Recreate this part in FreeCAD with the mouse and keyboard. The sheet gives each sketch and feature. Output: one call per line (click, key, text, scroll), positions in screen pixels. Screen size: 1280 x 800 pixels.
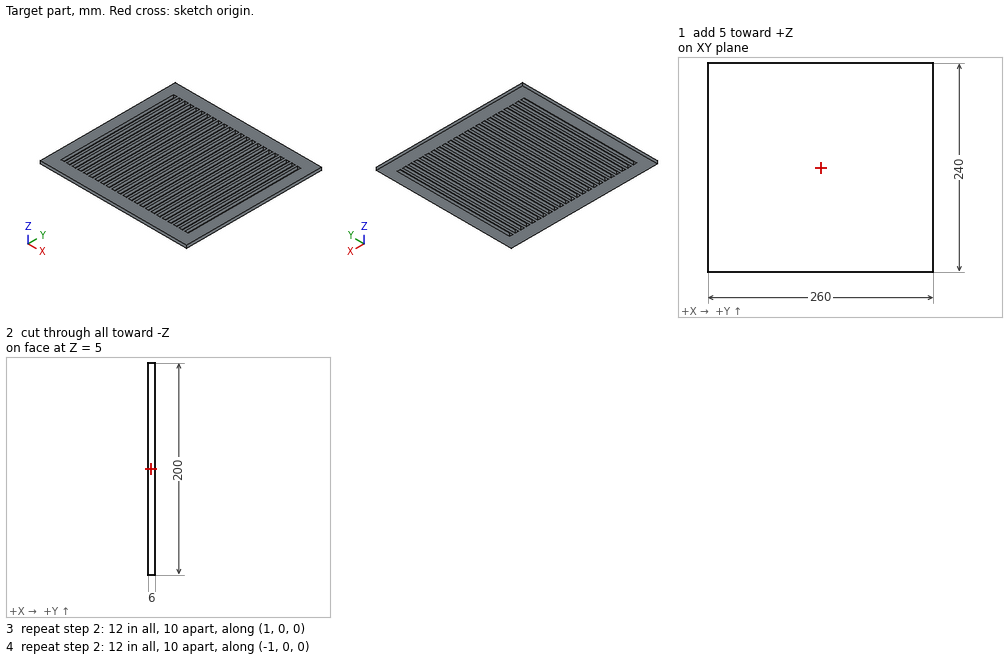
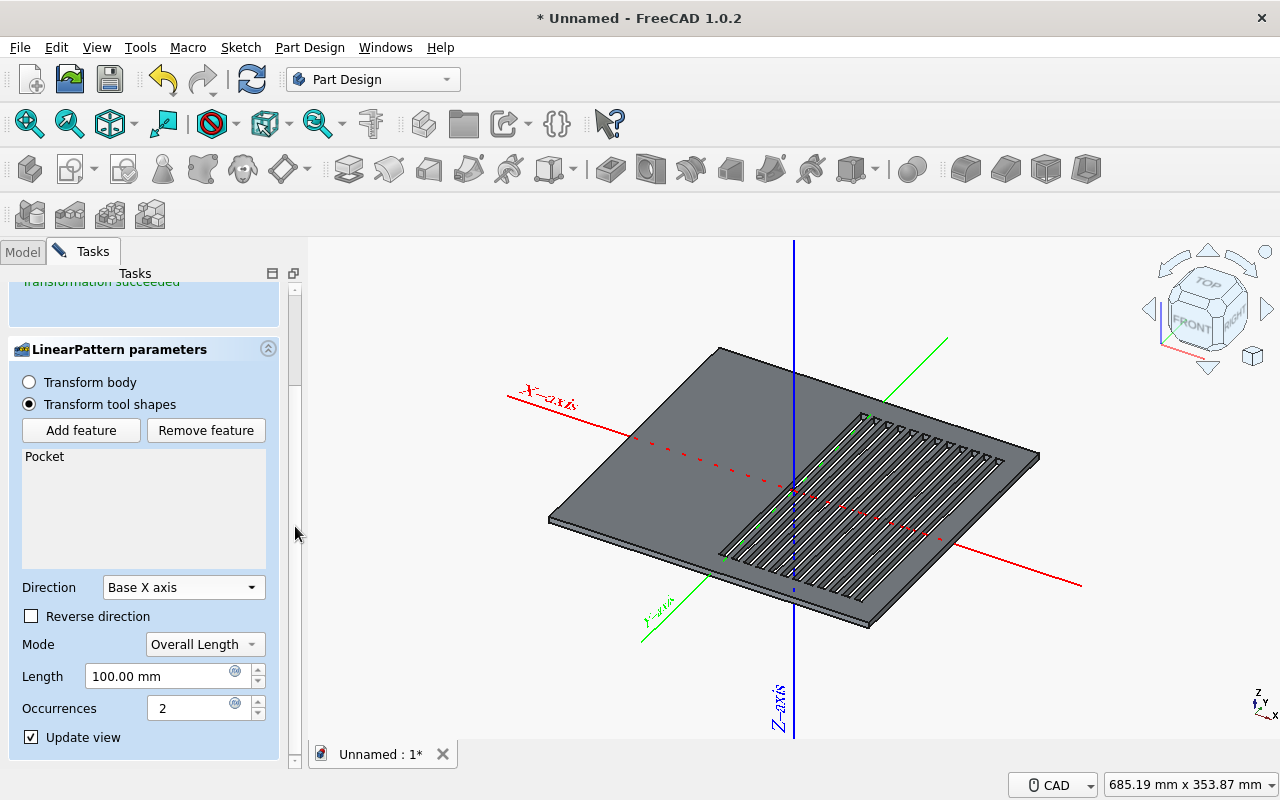
click(206, 644)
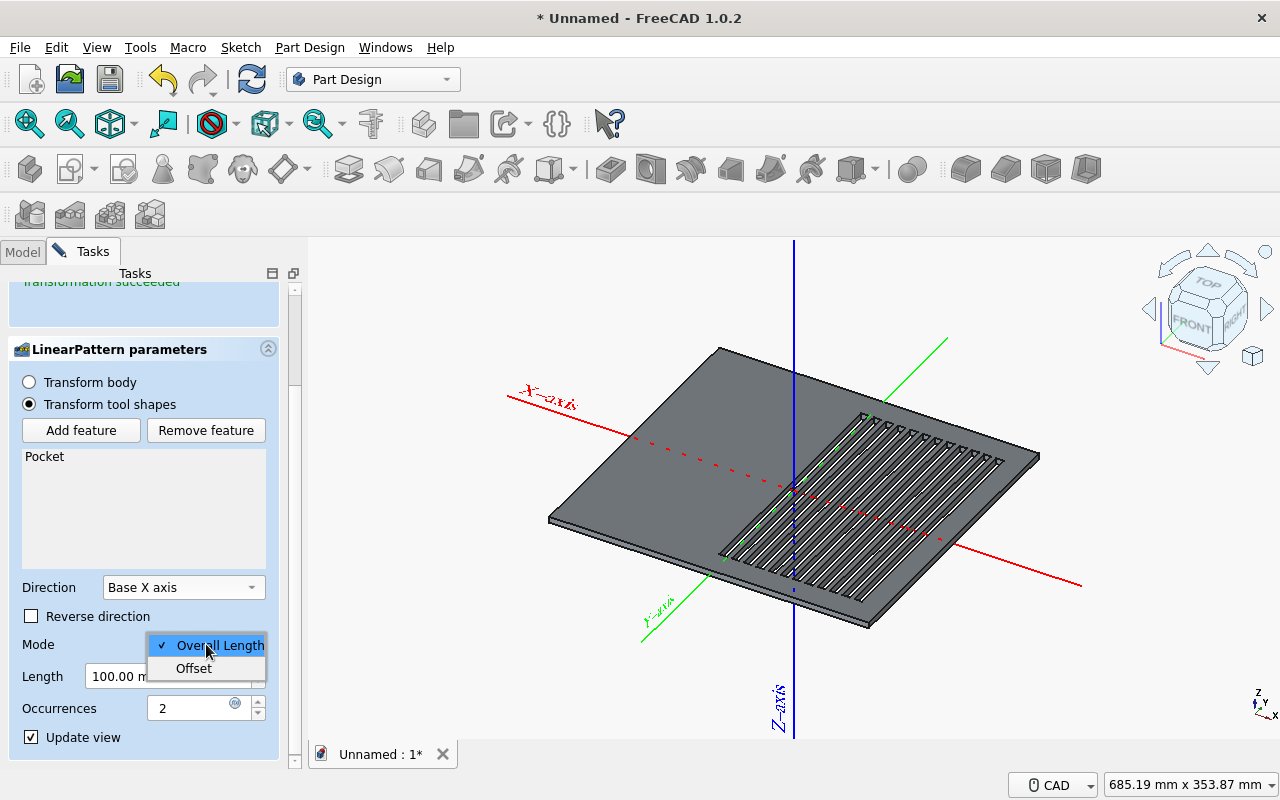
click(206, 668)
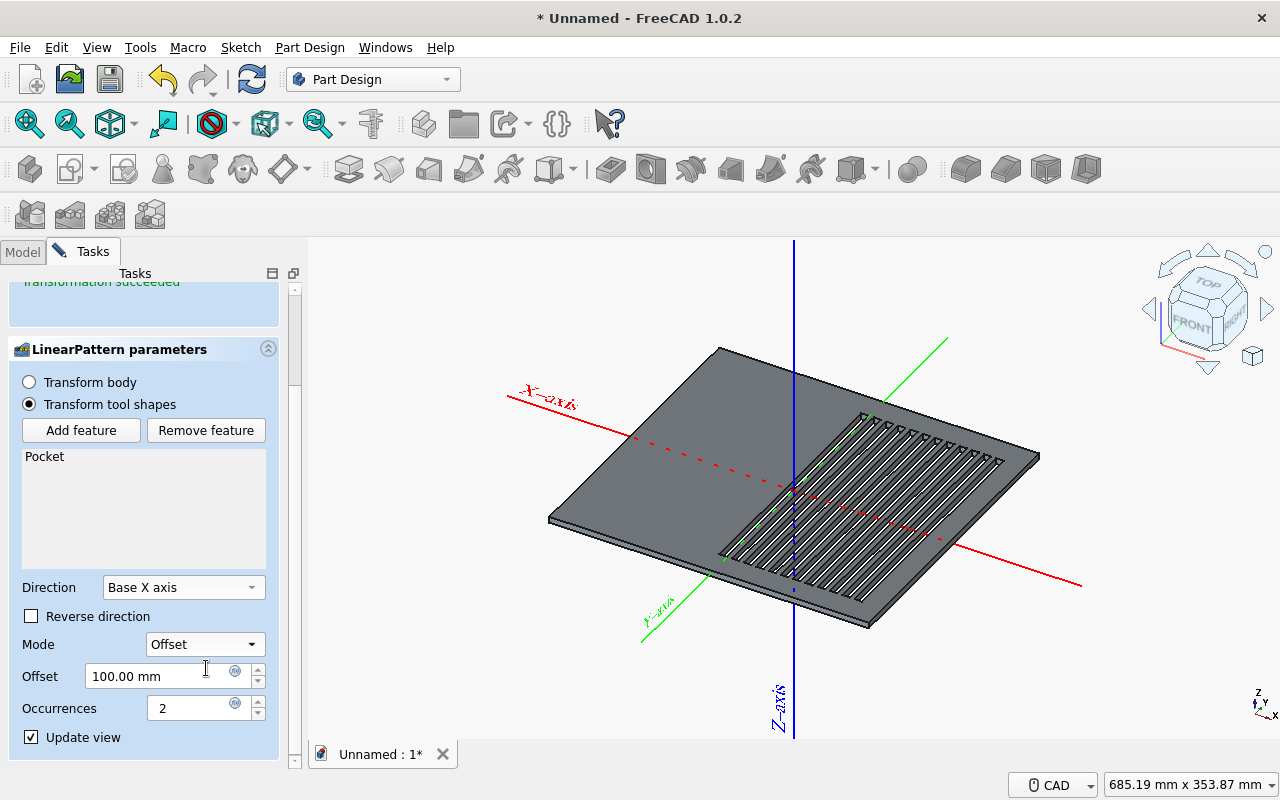
triple_click(168, 676)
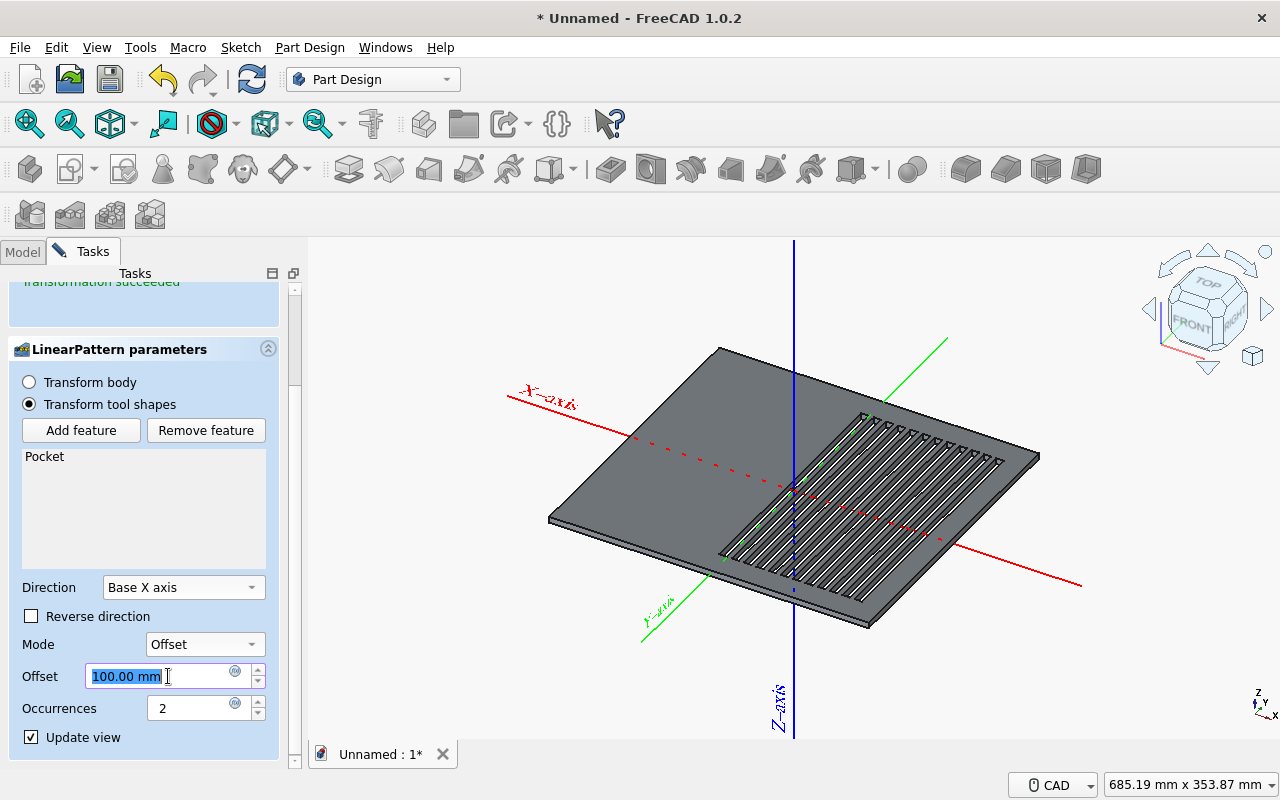
text(10)
key(Tab)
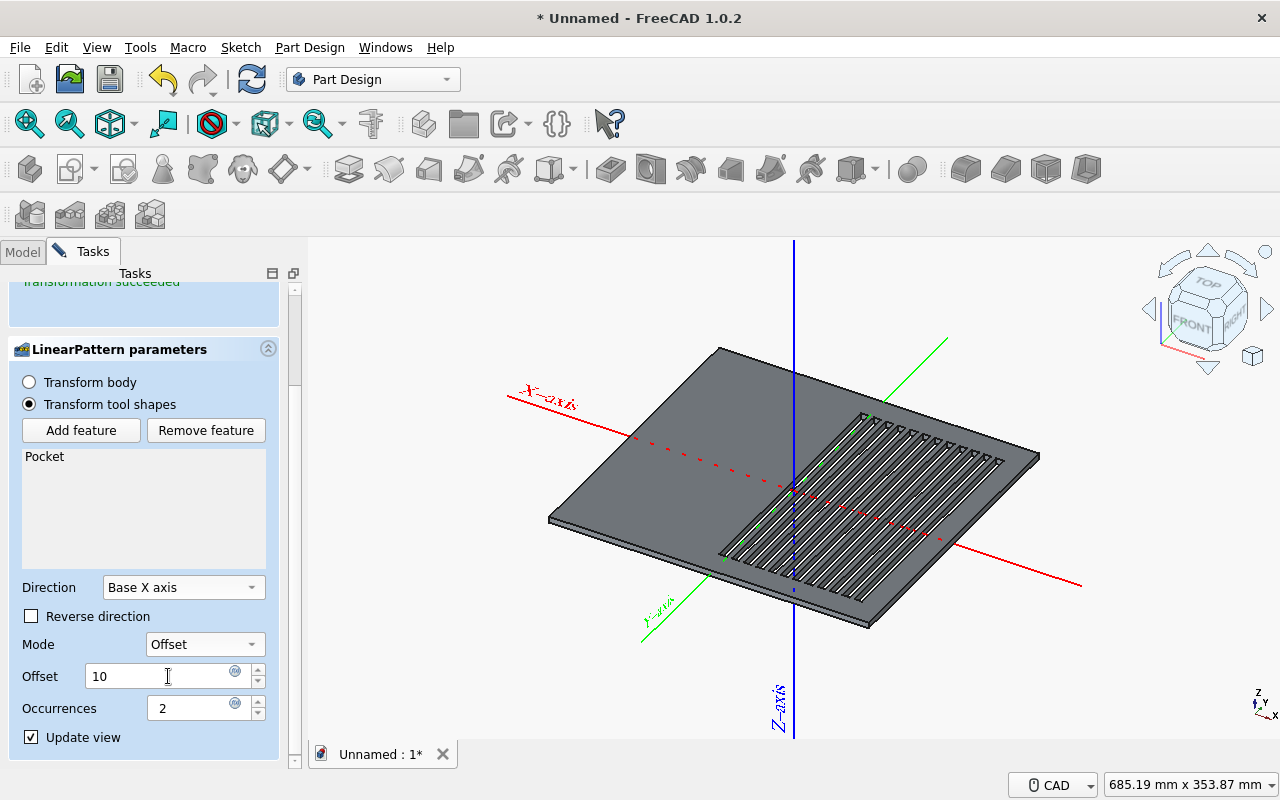
triple_click(198, 708)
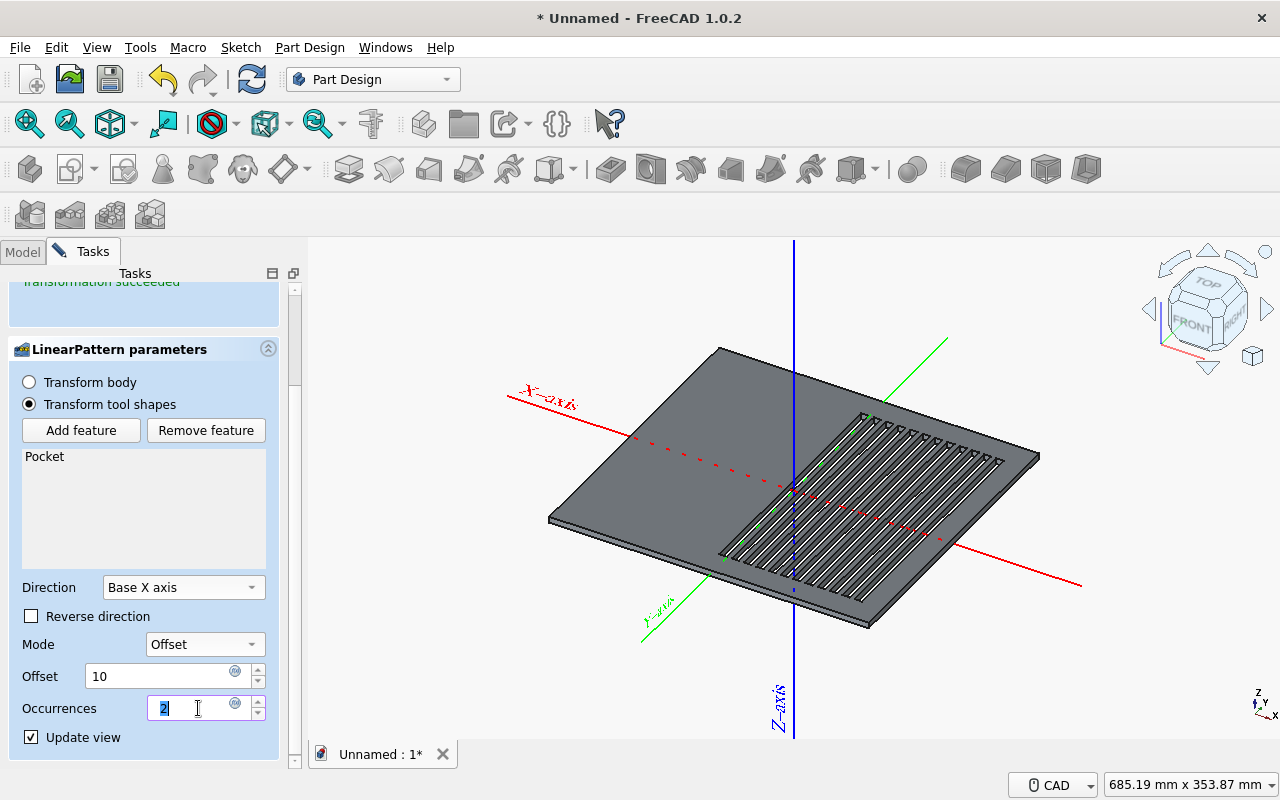
text(12)
key(Tab)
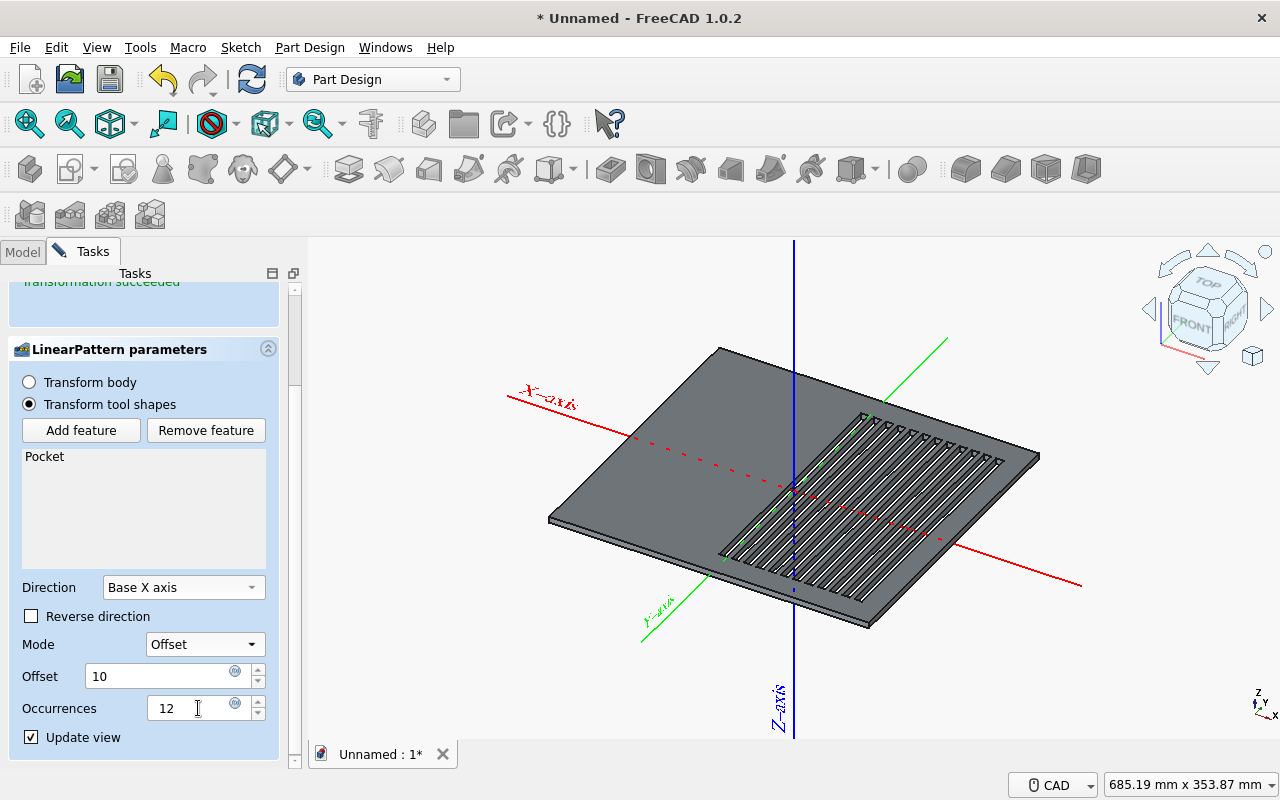
click(30, 616)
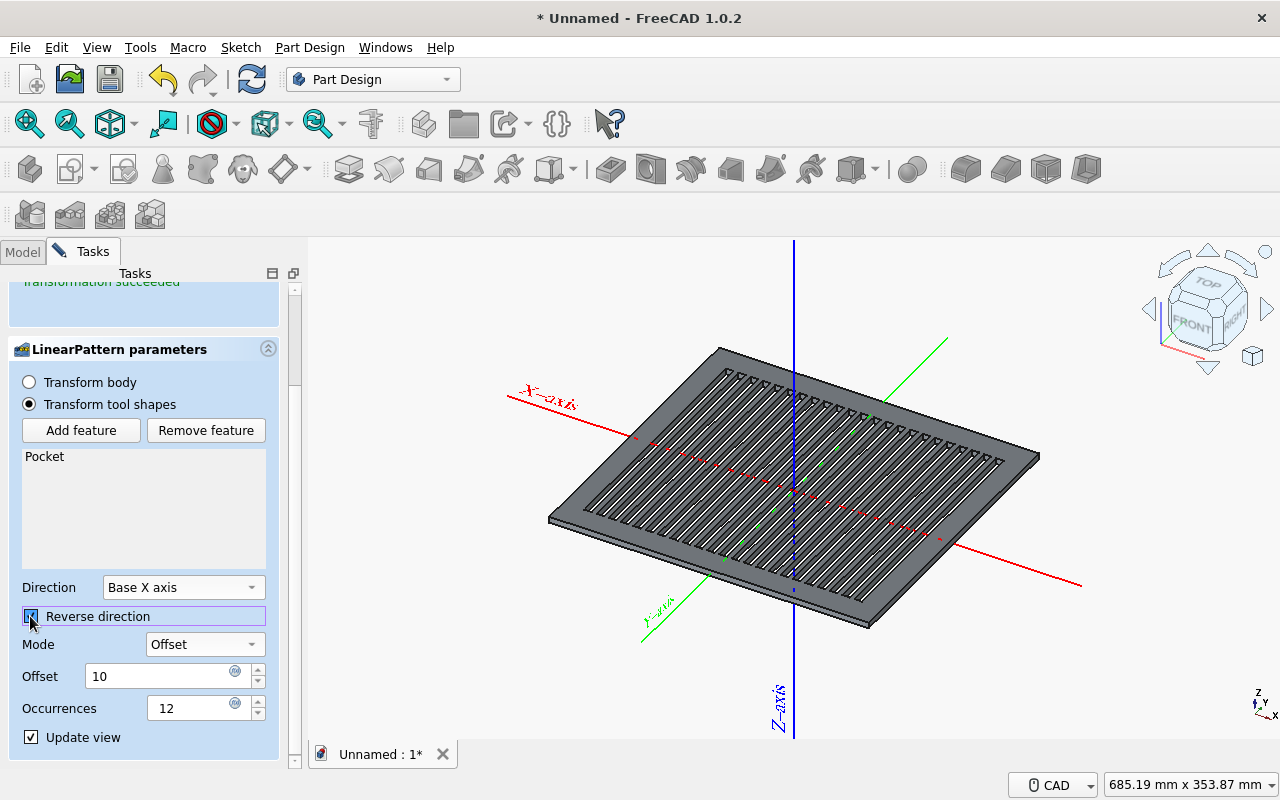
scroll(295, 526, up, 3)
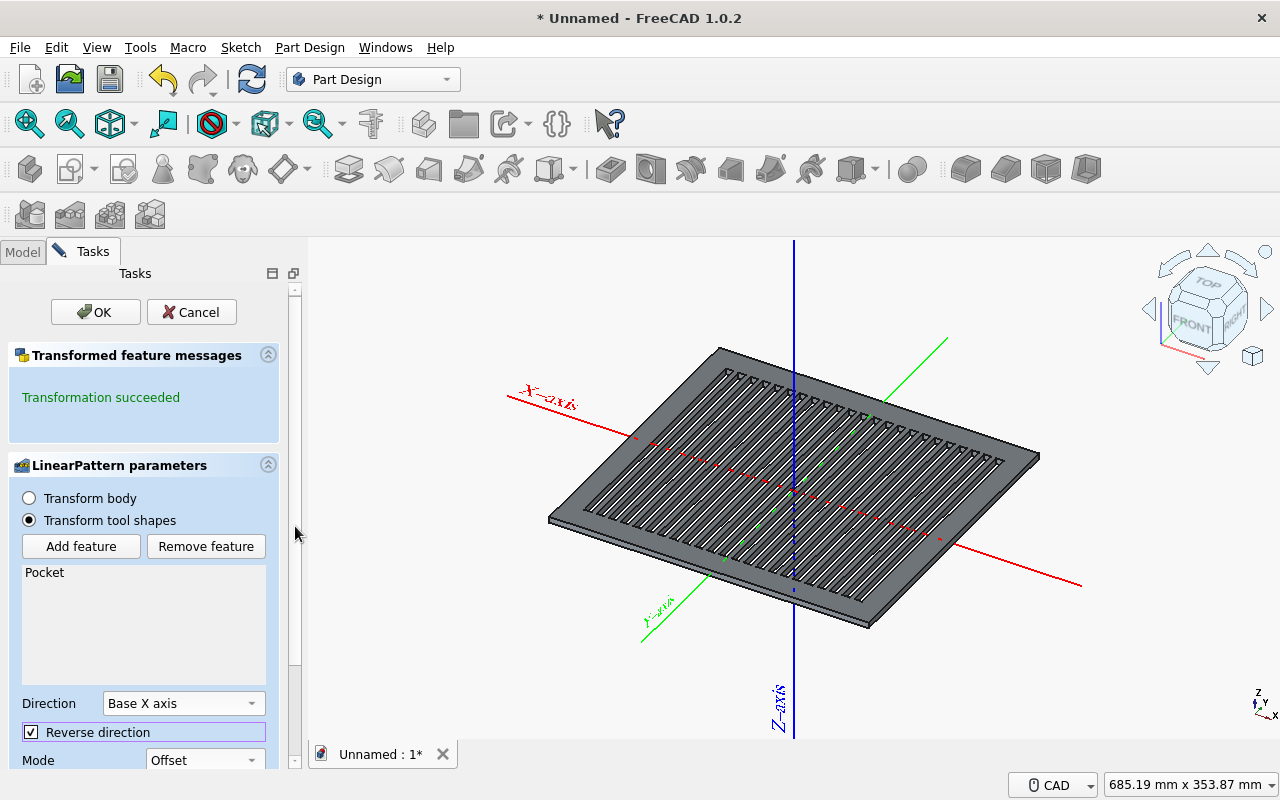
click(96, 312)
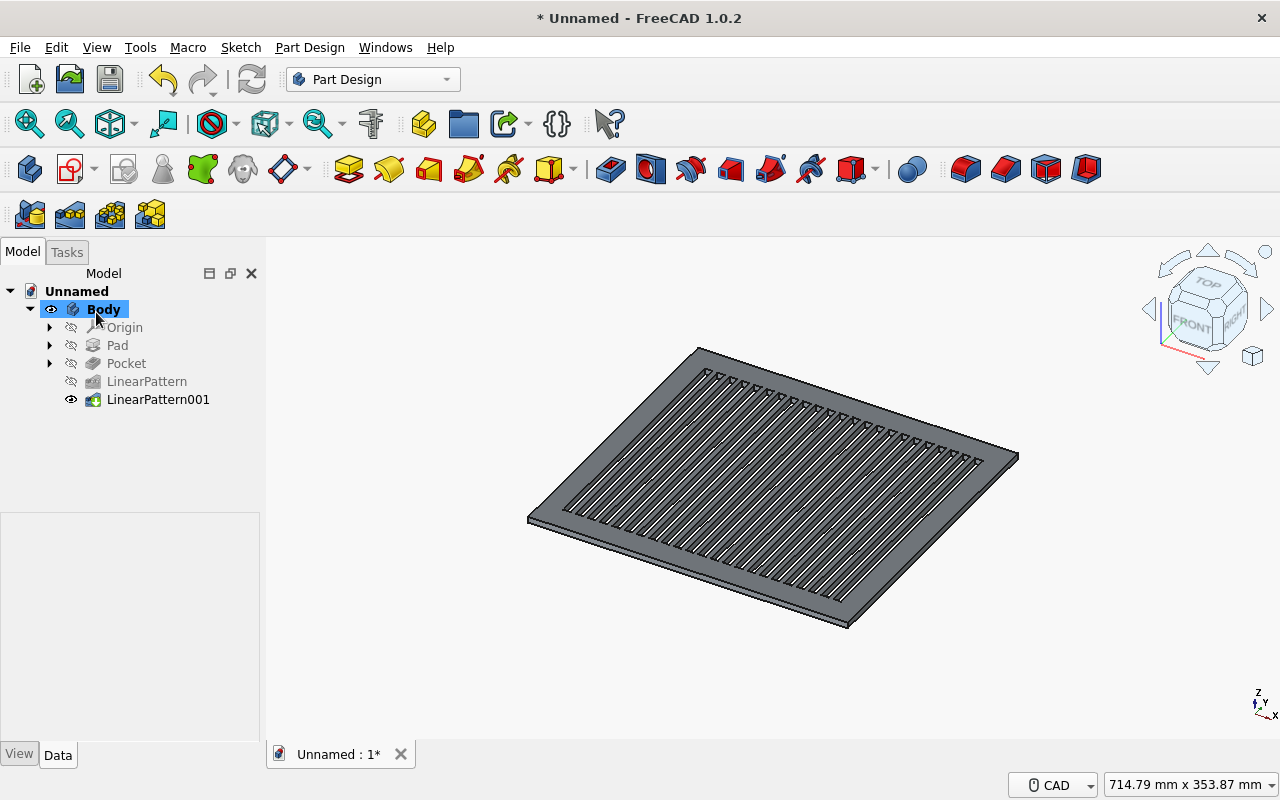
key(0)